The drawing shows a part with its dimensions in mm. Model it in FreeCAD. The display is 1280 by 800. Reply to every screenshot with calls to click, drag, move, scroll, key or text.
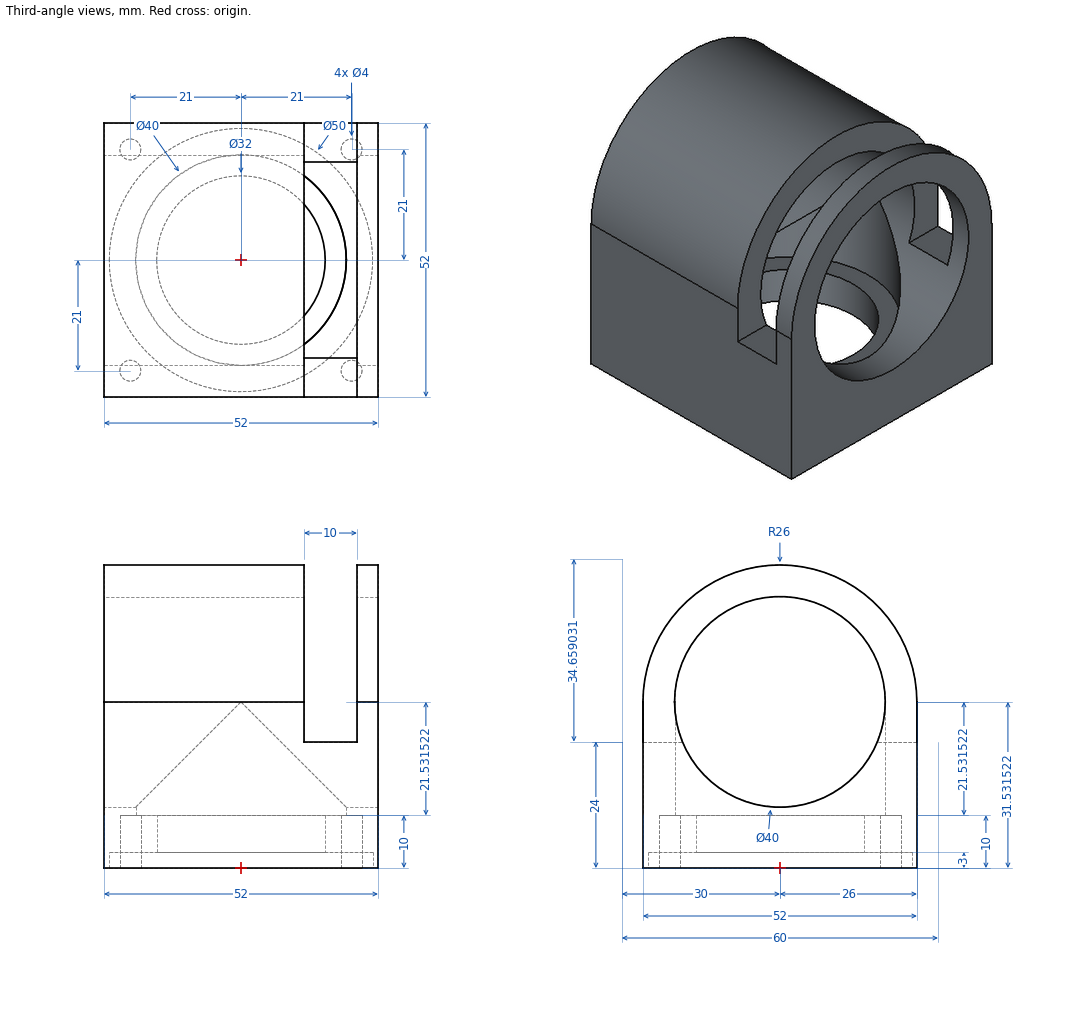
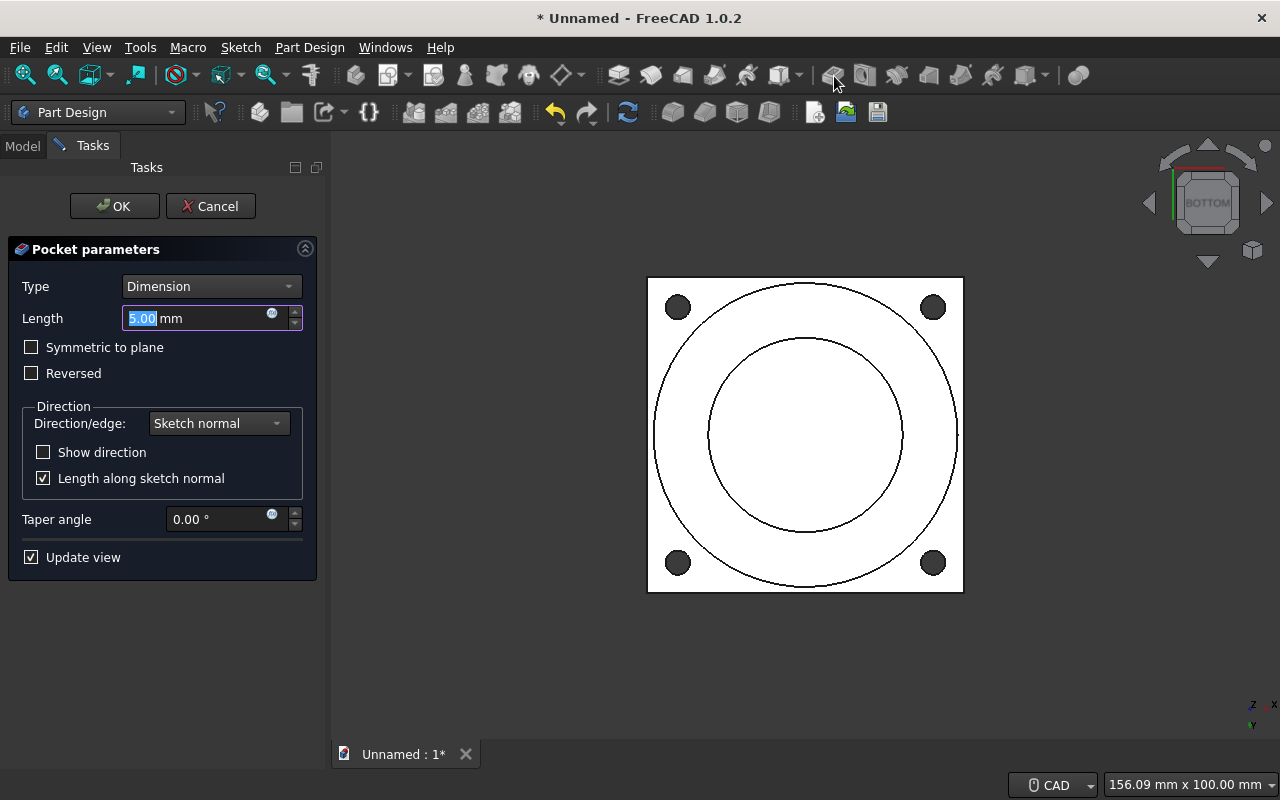
click(212, 286)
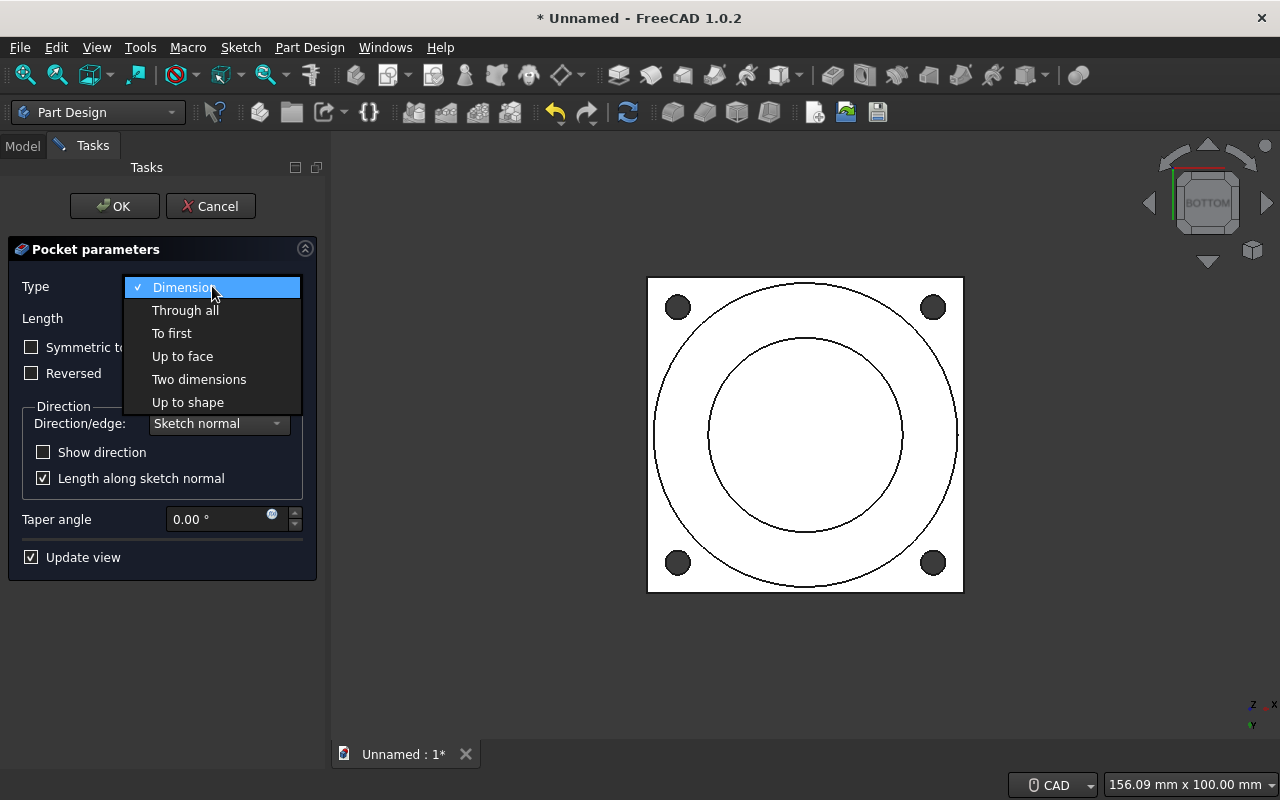
click(212, 310)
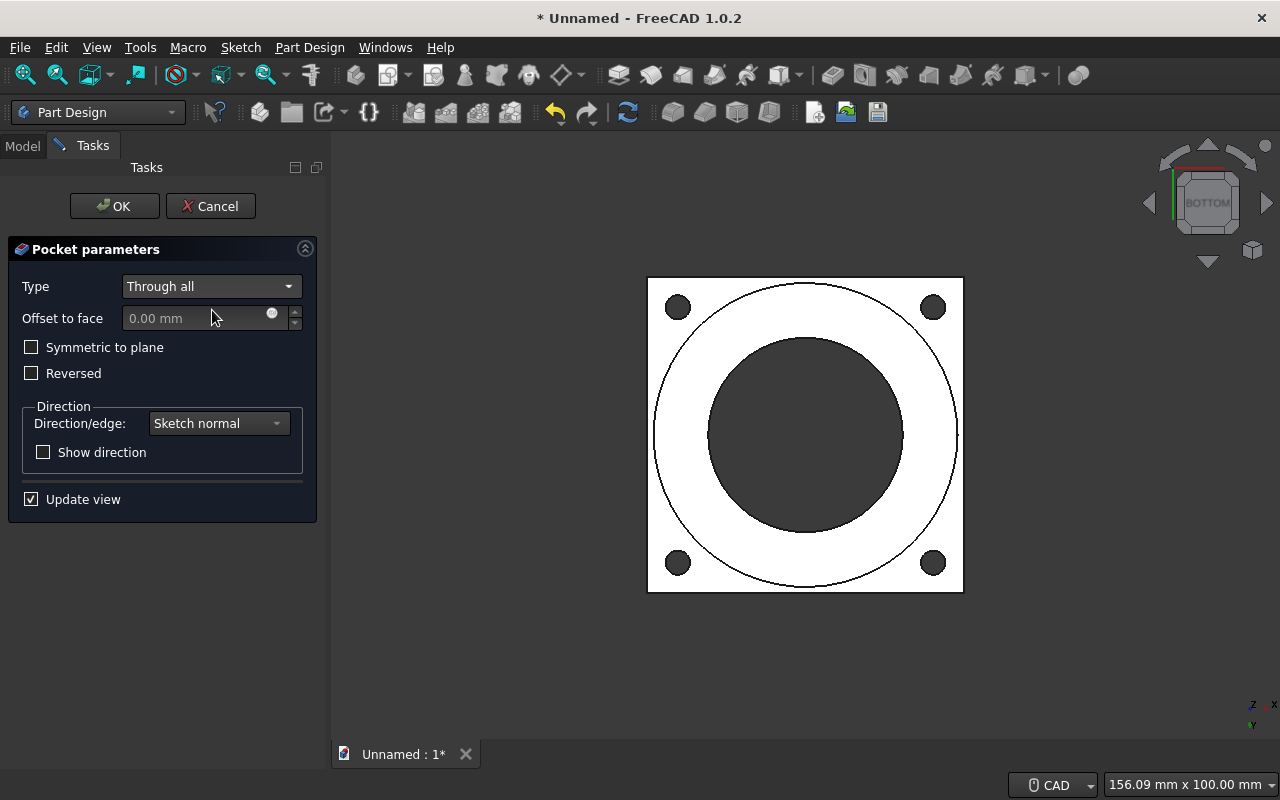
click(115, 206)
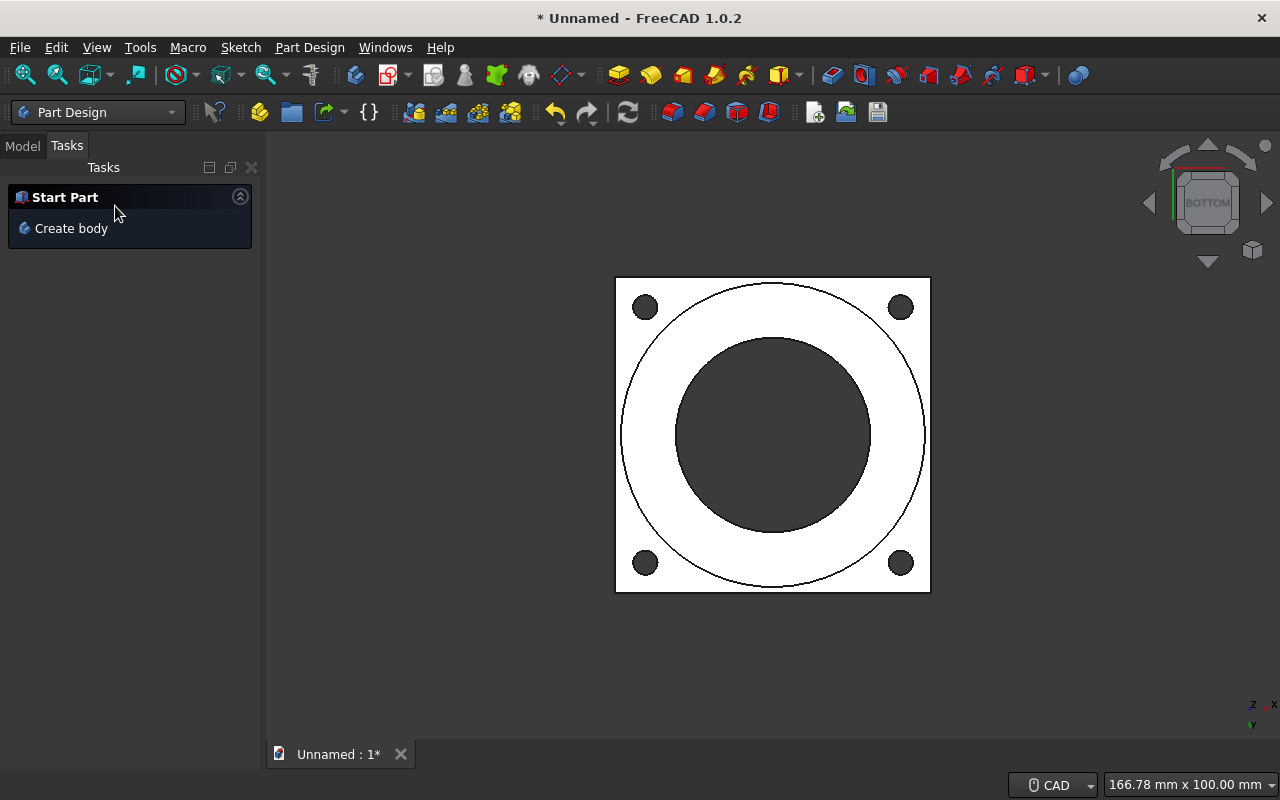
key(6)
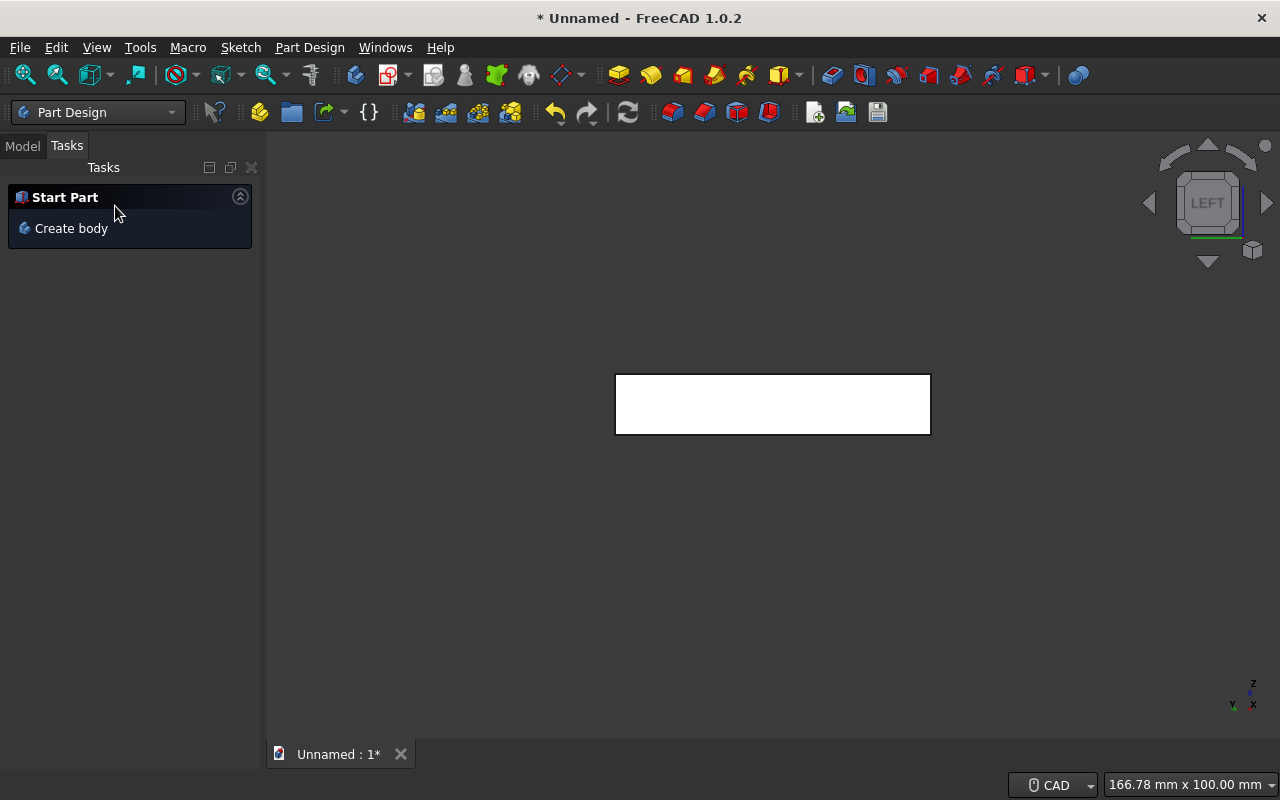
click(26, 76)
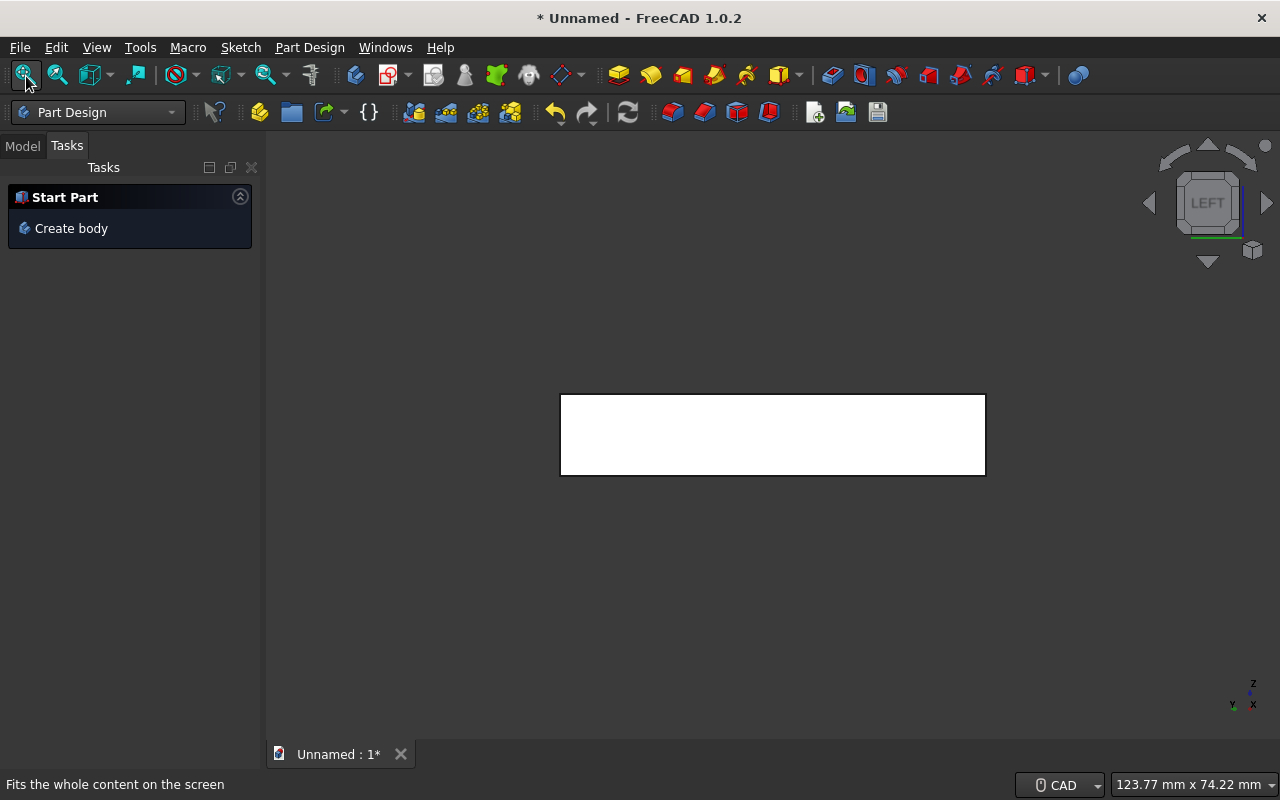
click(651, 434)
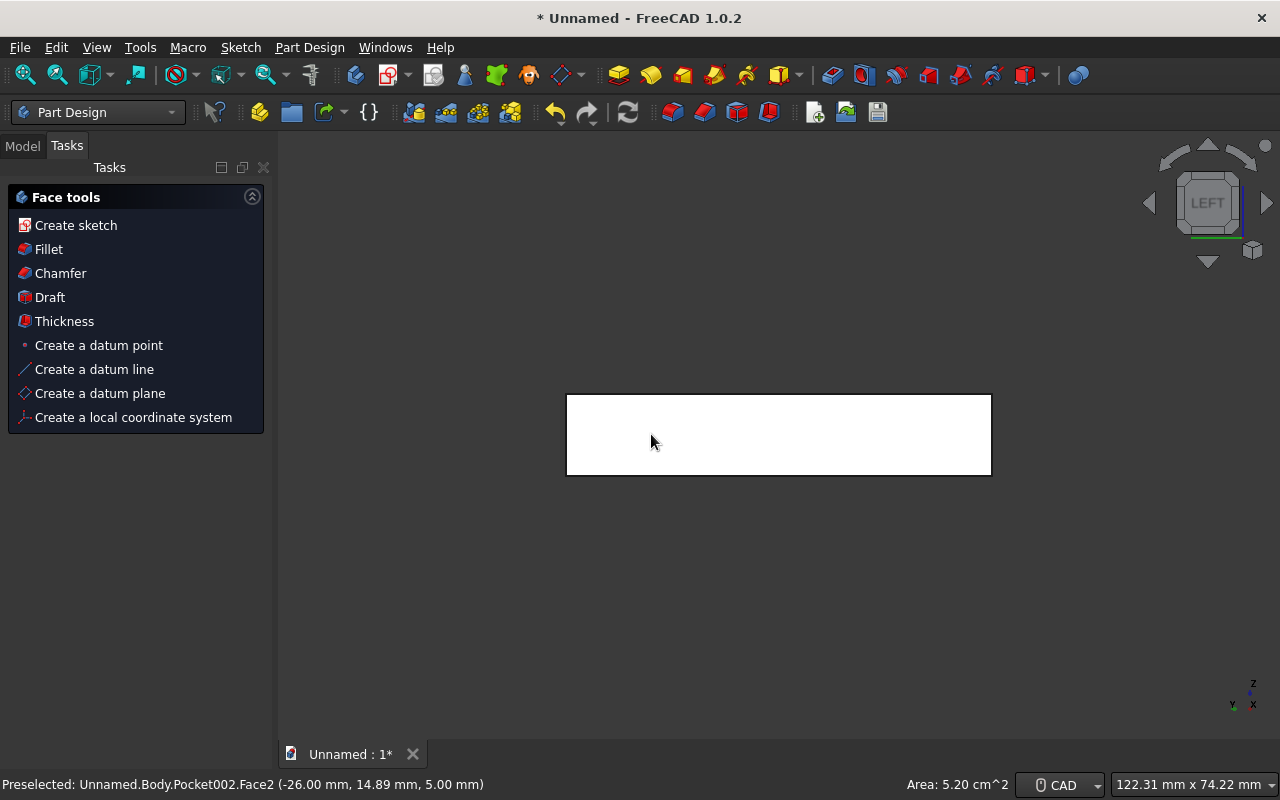
click(388, 76)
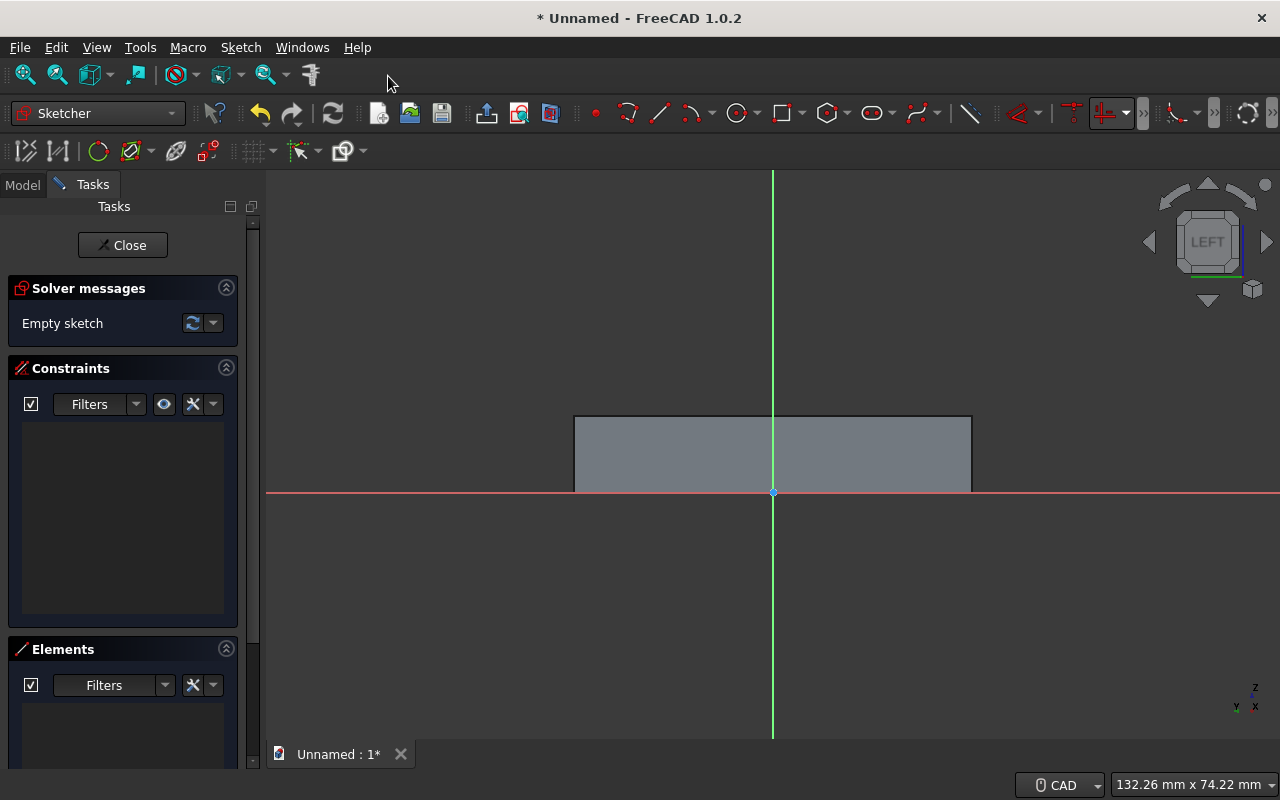
scroll(912, 204, up, 2)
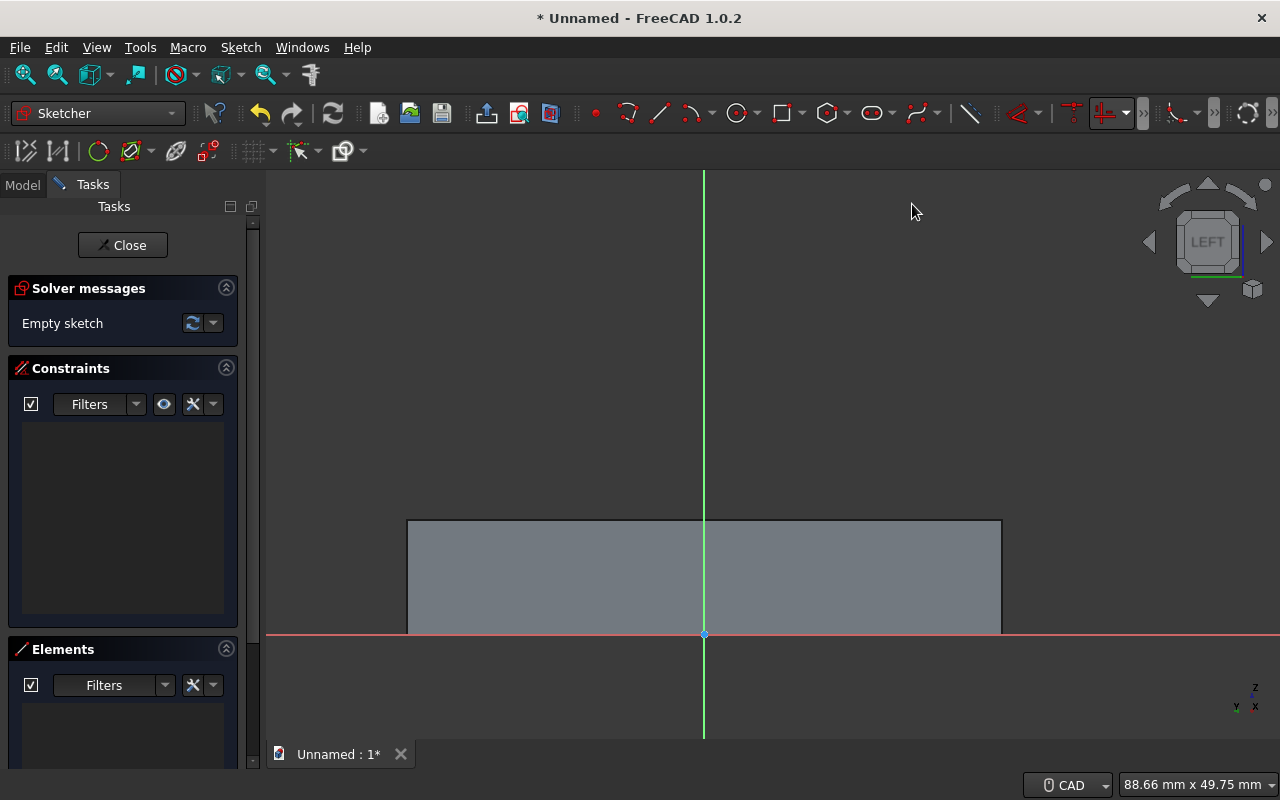
click(782, 114)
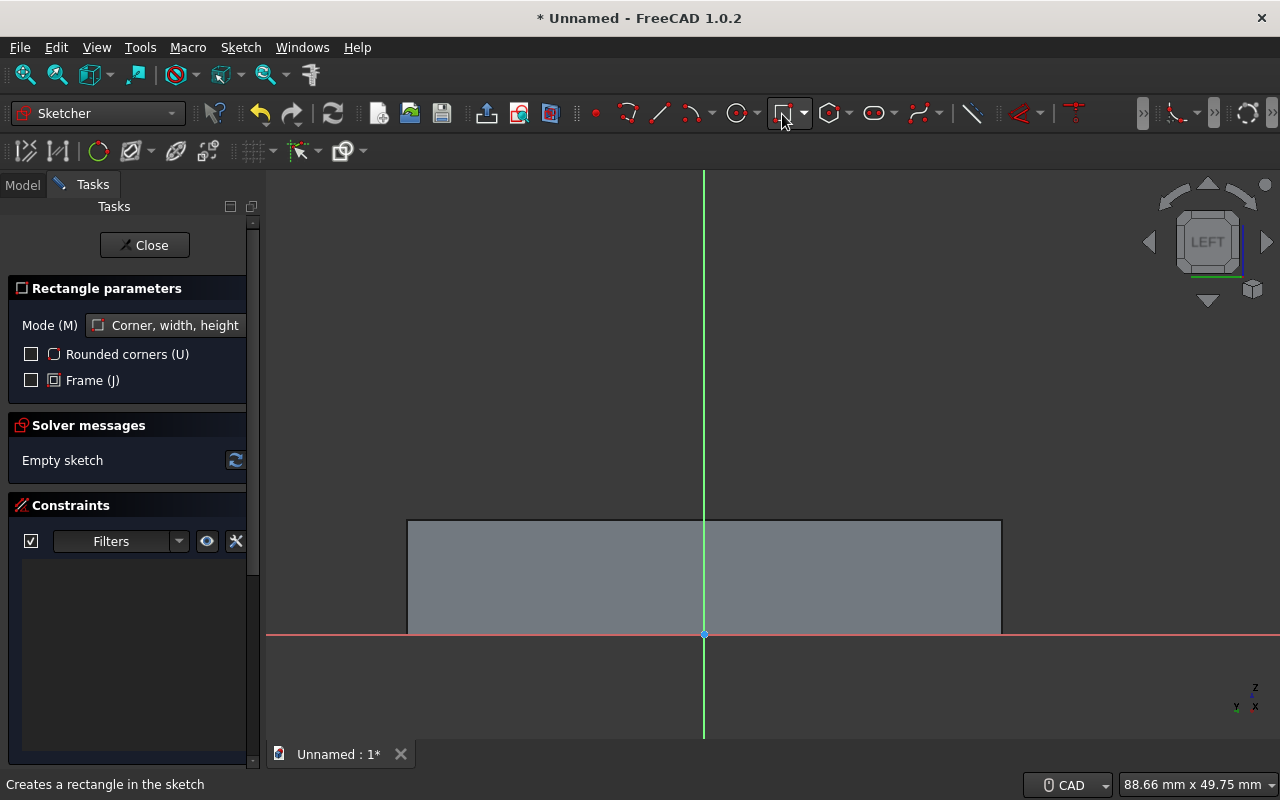
click(407, 274)
click(1002, 520)
key(Escape)